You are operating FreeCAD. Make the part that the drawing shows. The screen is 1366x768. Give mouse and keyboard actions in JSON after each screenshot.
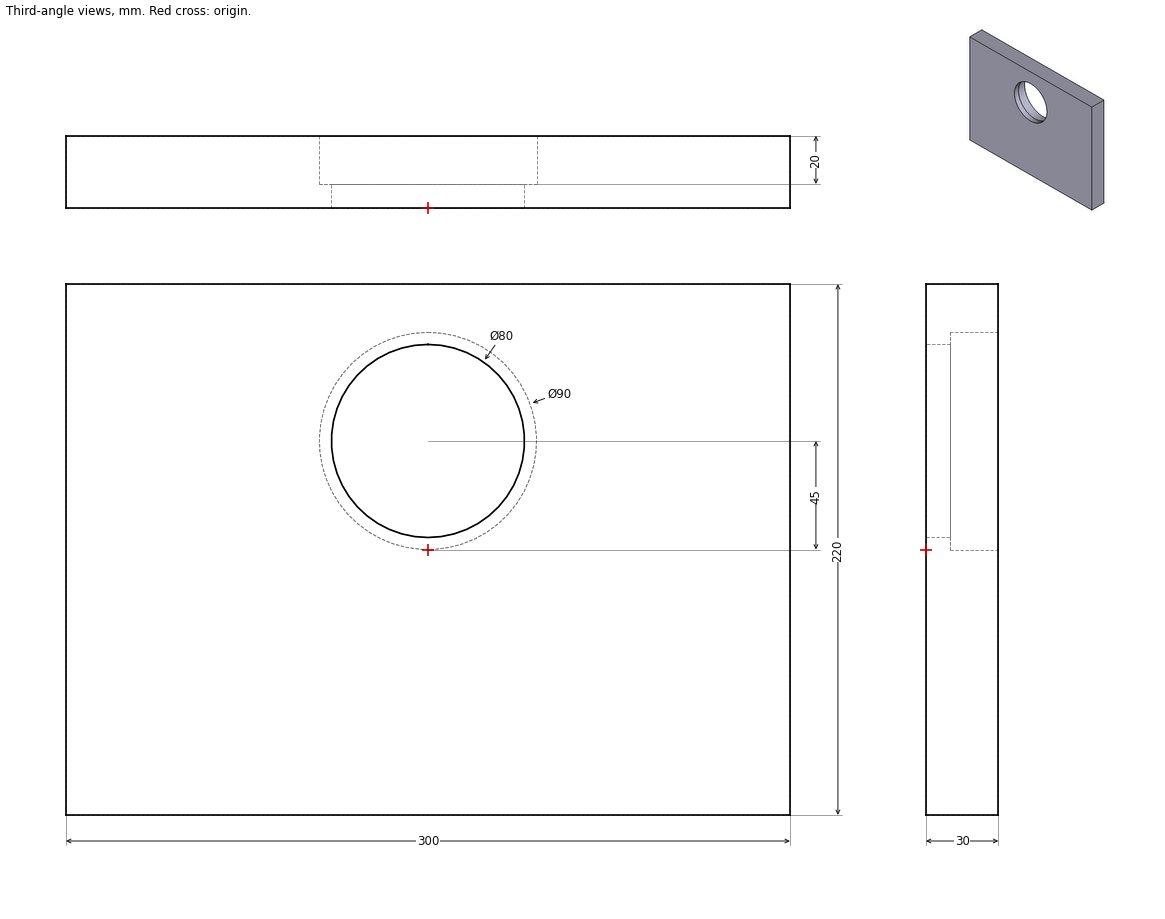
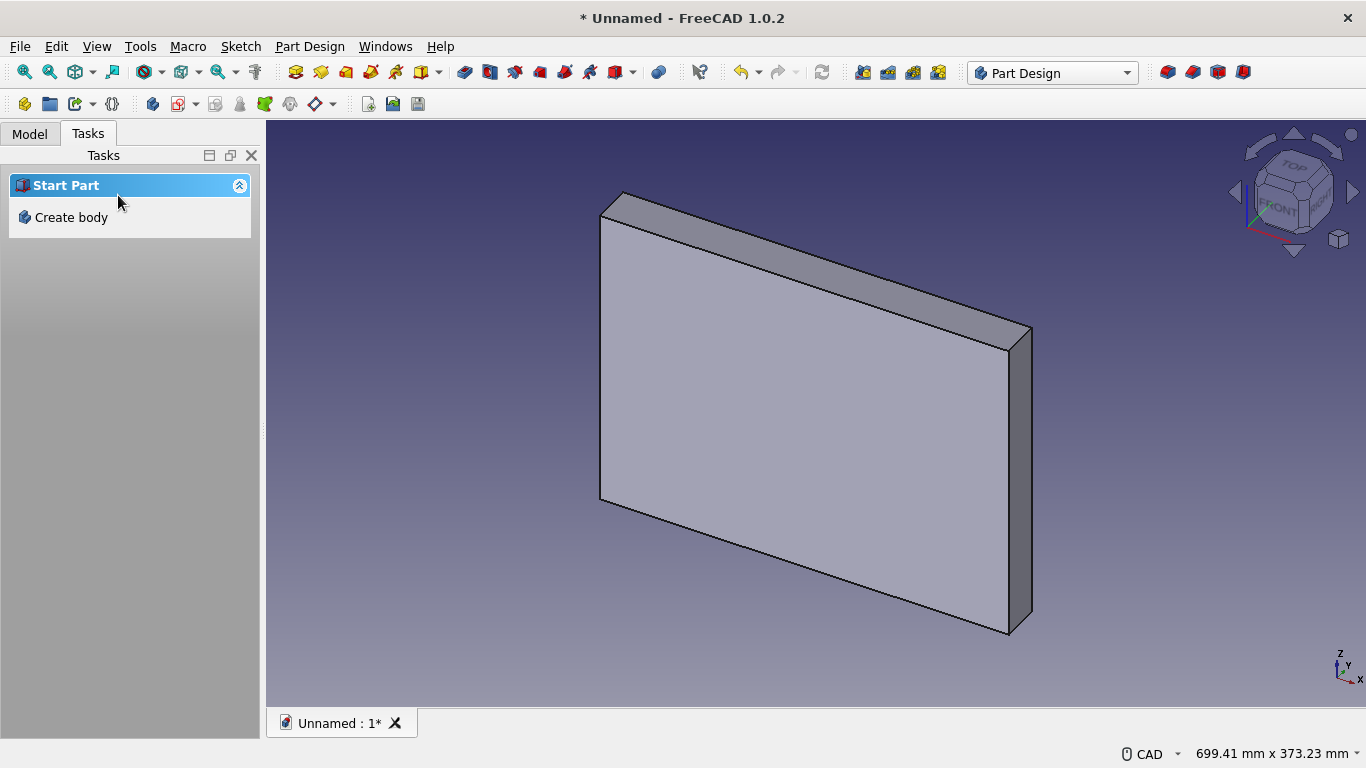
{"action": "key", "text": "4"}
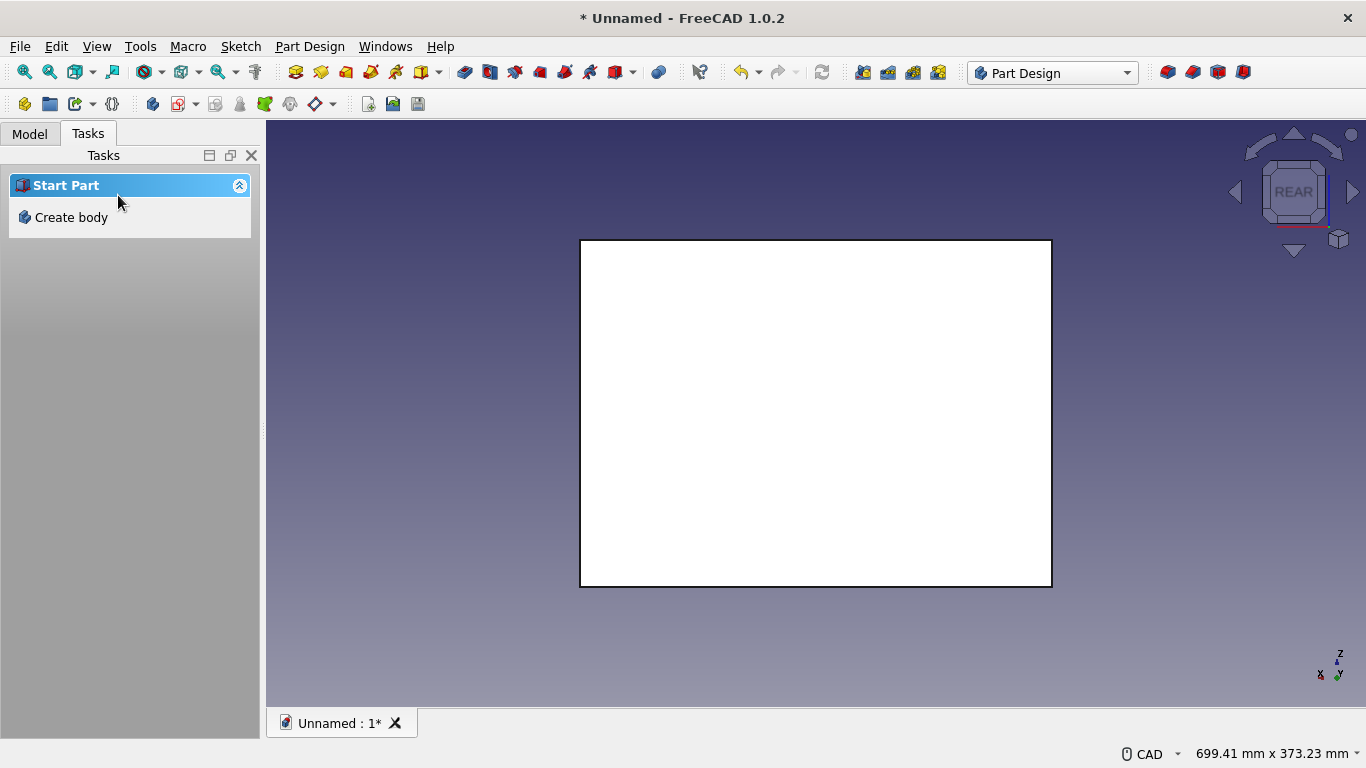
{"action": "left_click", "coordinate": [816, 413]}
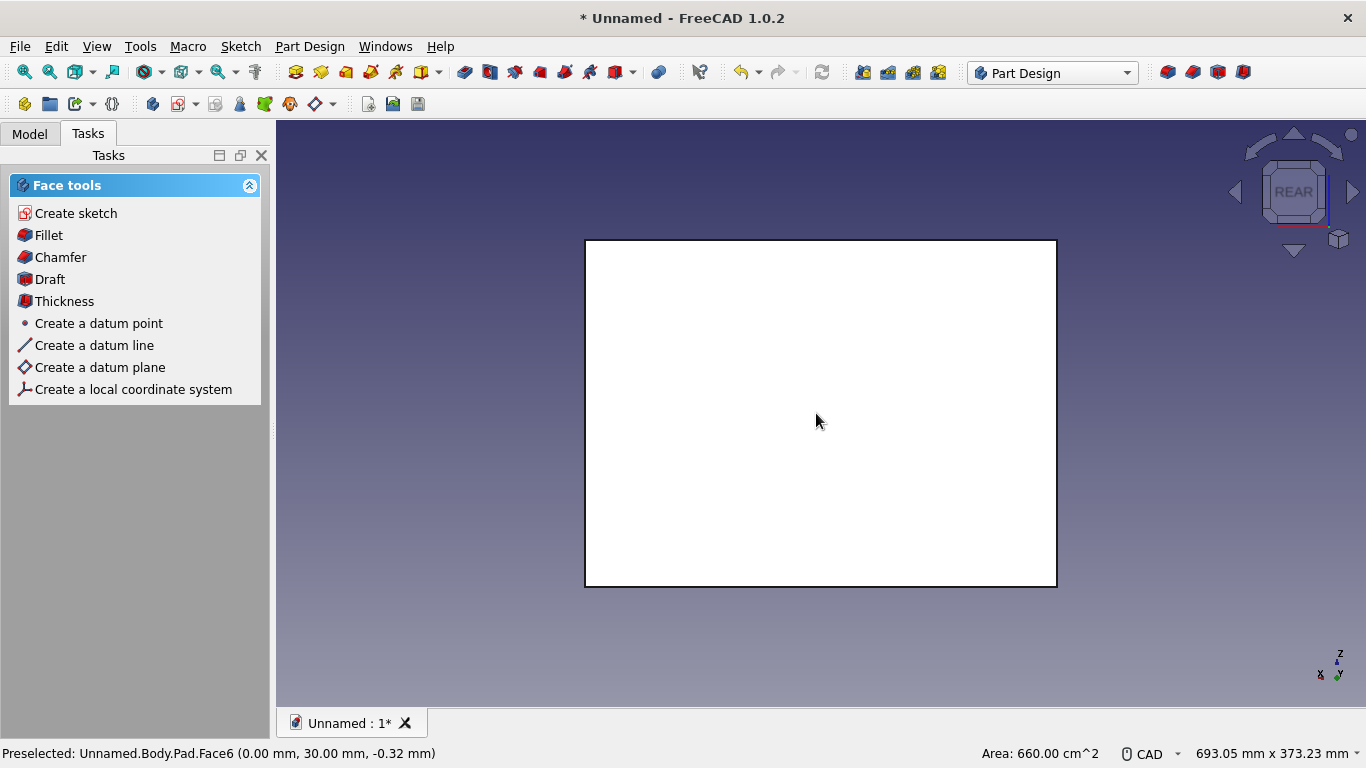
{"action": "left_click", "coordinate": [178, 104]}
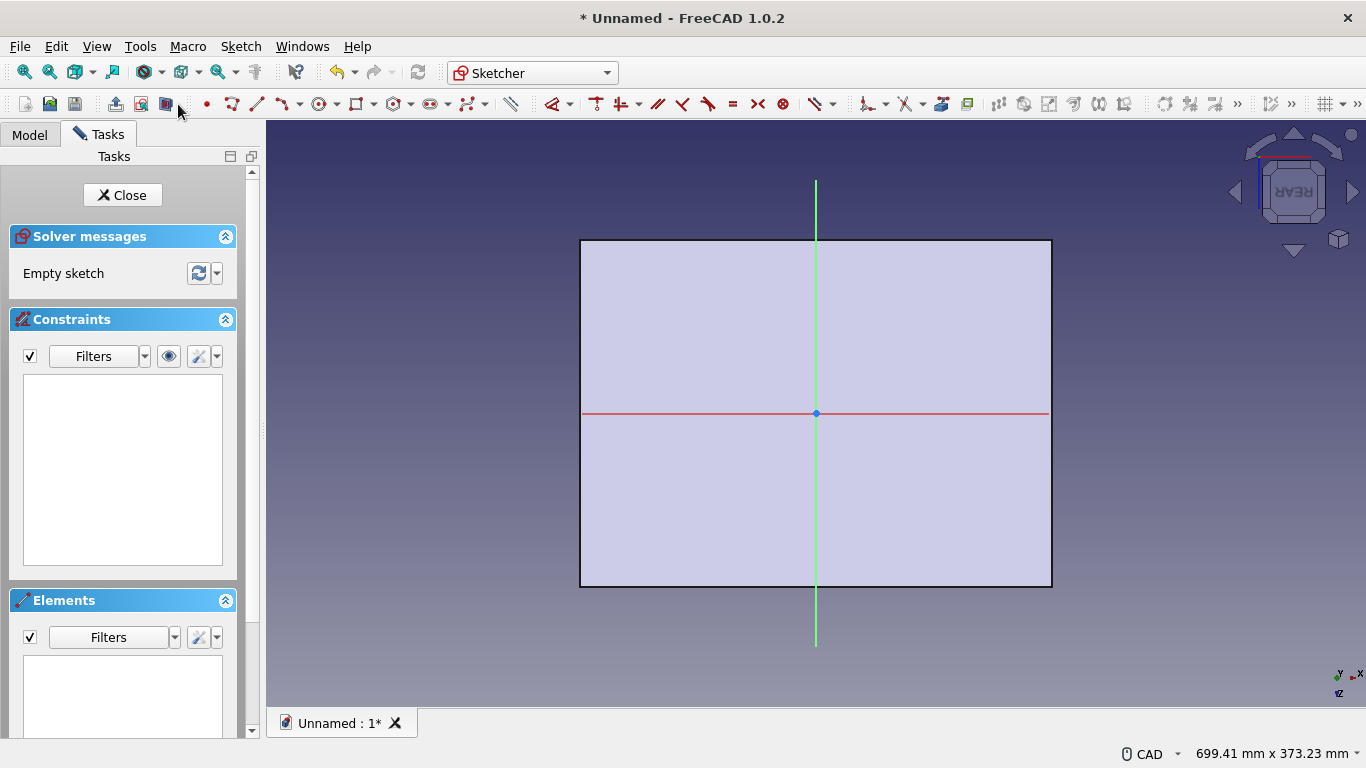
{"action": "scroll", "coordinate": [856, 525], "scroll_direction": "up", "scroll_amount": 5}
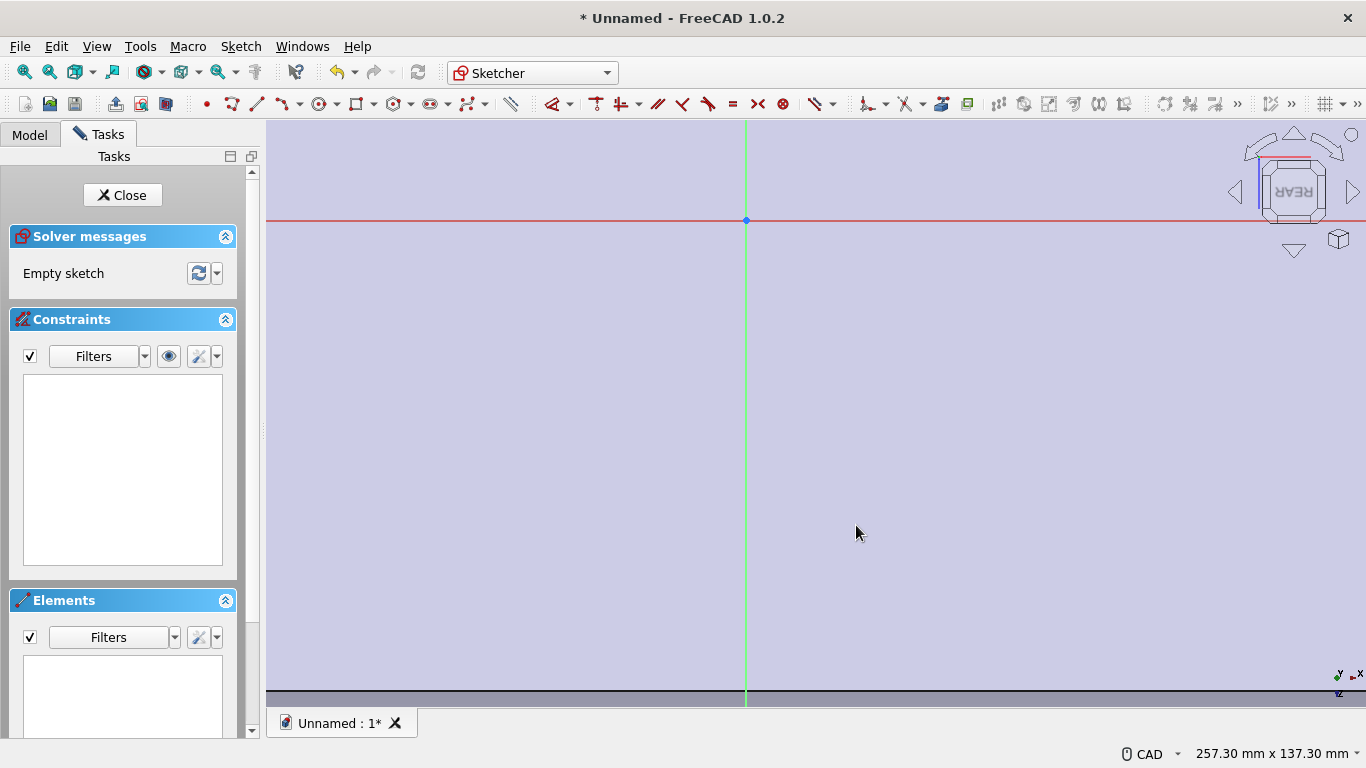
{"action": "left_click", "coordinate": [318, 104]}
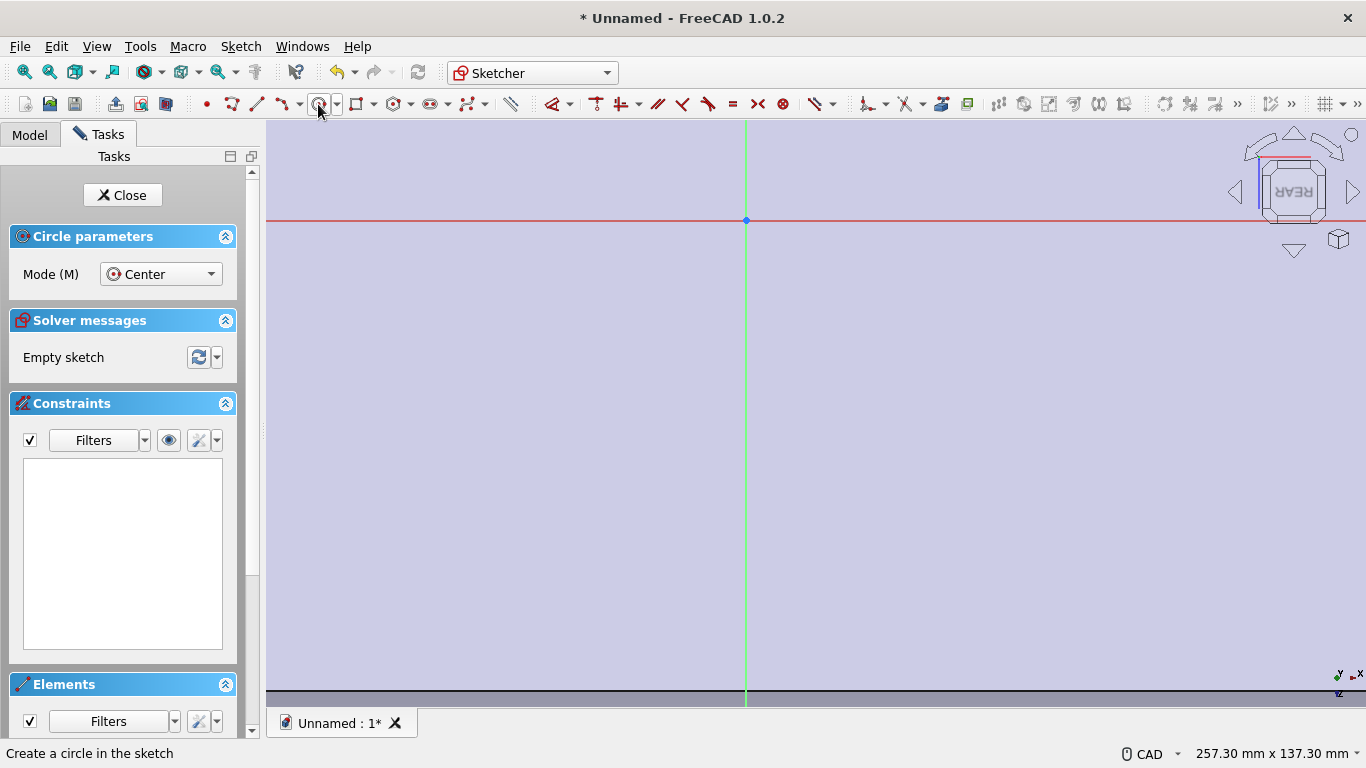
{"action": "left_click", "coordinate": [746, 413]}
{"action": "left_click", "coordinate": [882, 277]}
{"action": "key", "text": "Escape"}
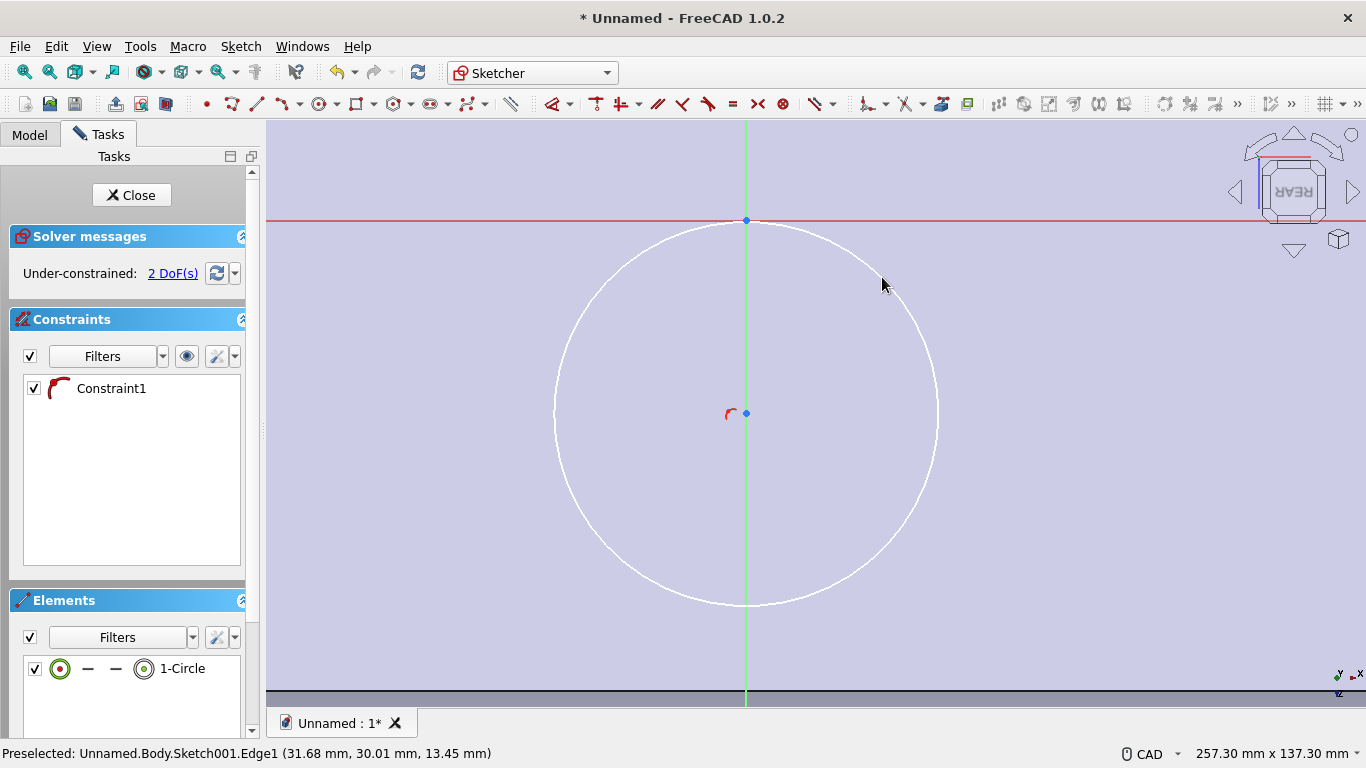
{"action": "key", "text": "d"}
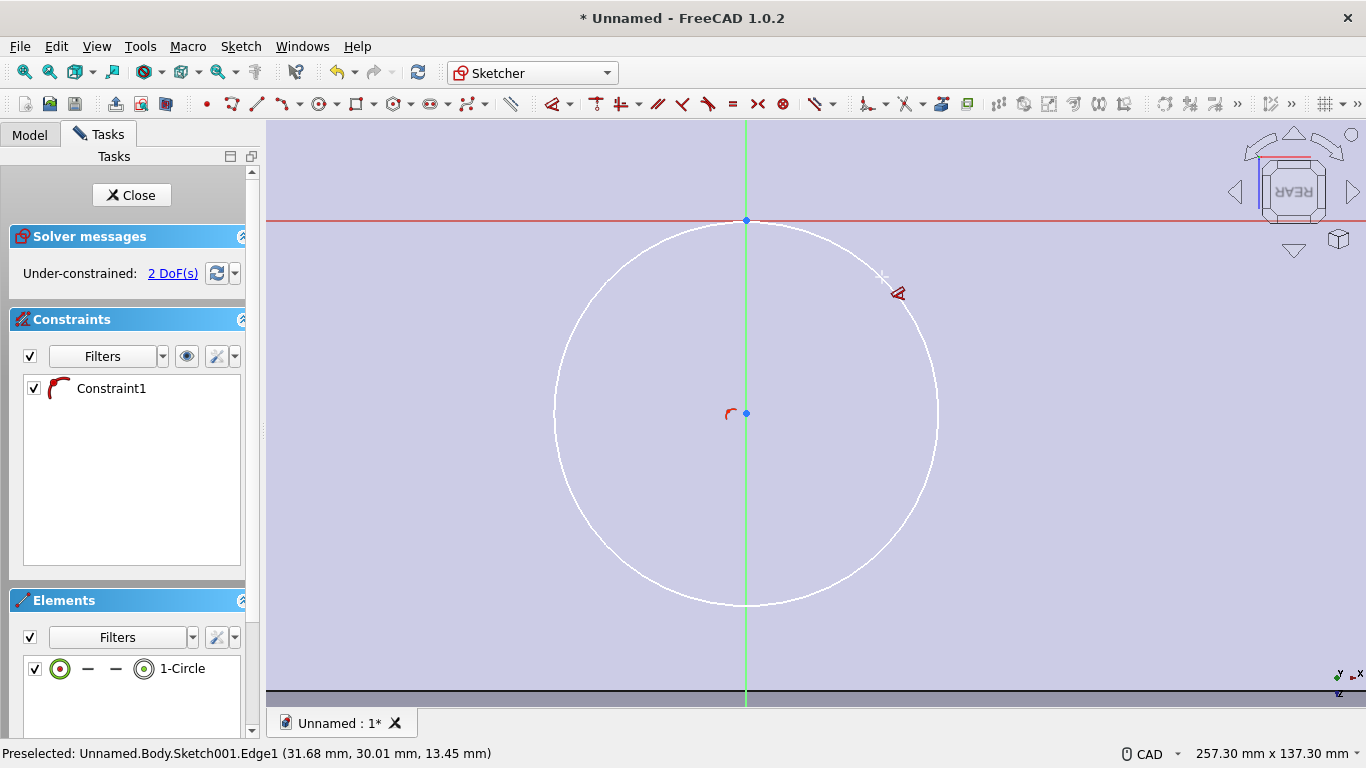
{"action": "left_click", "coordinate": [882, 278]}
{"action": "left_click", "coordinate": [905, 255]}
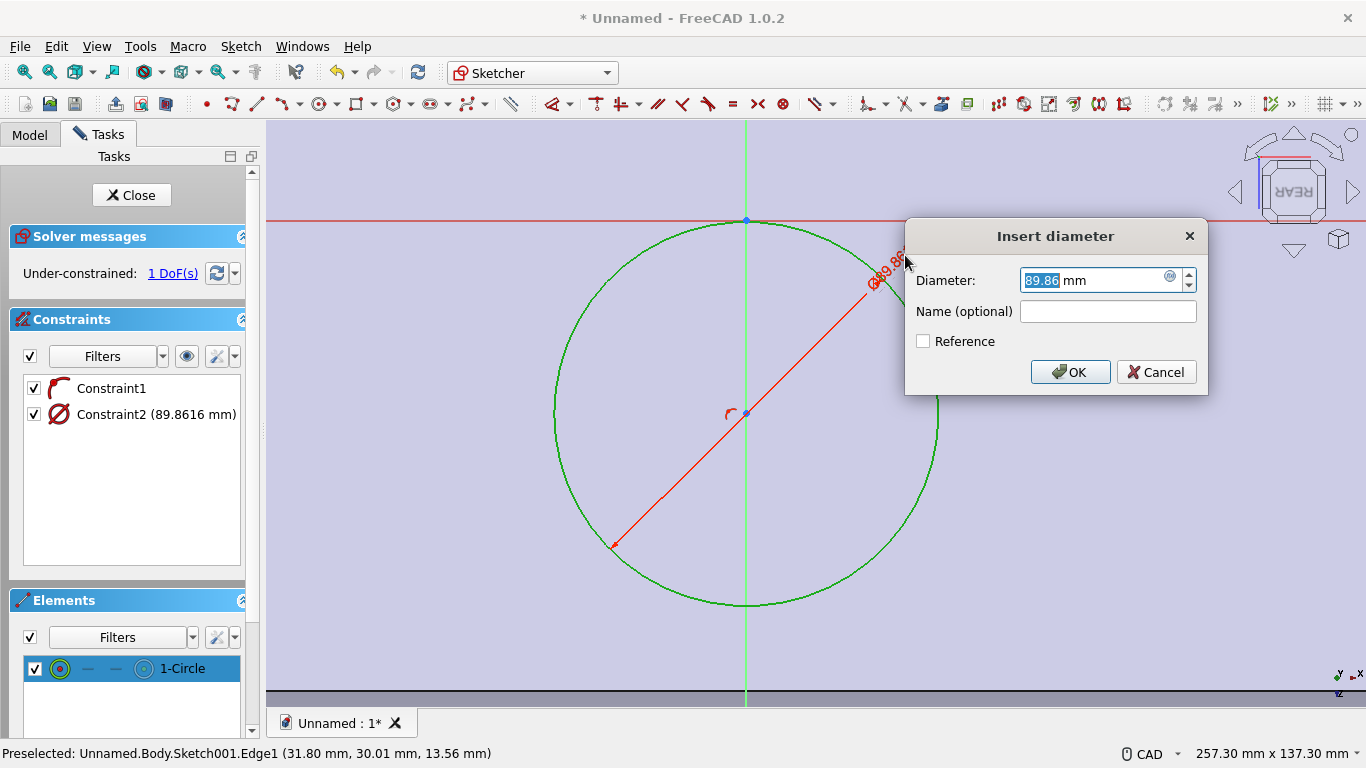
{"action": "type", "text": "90"}
{"action": "key", "text": "Return"}